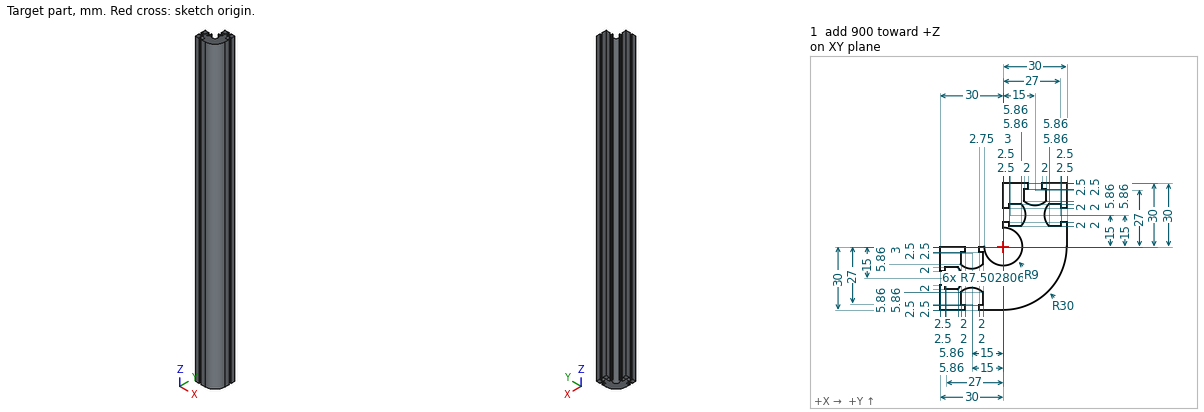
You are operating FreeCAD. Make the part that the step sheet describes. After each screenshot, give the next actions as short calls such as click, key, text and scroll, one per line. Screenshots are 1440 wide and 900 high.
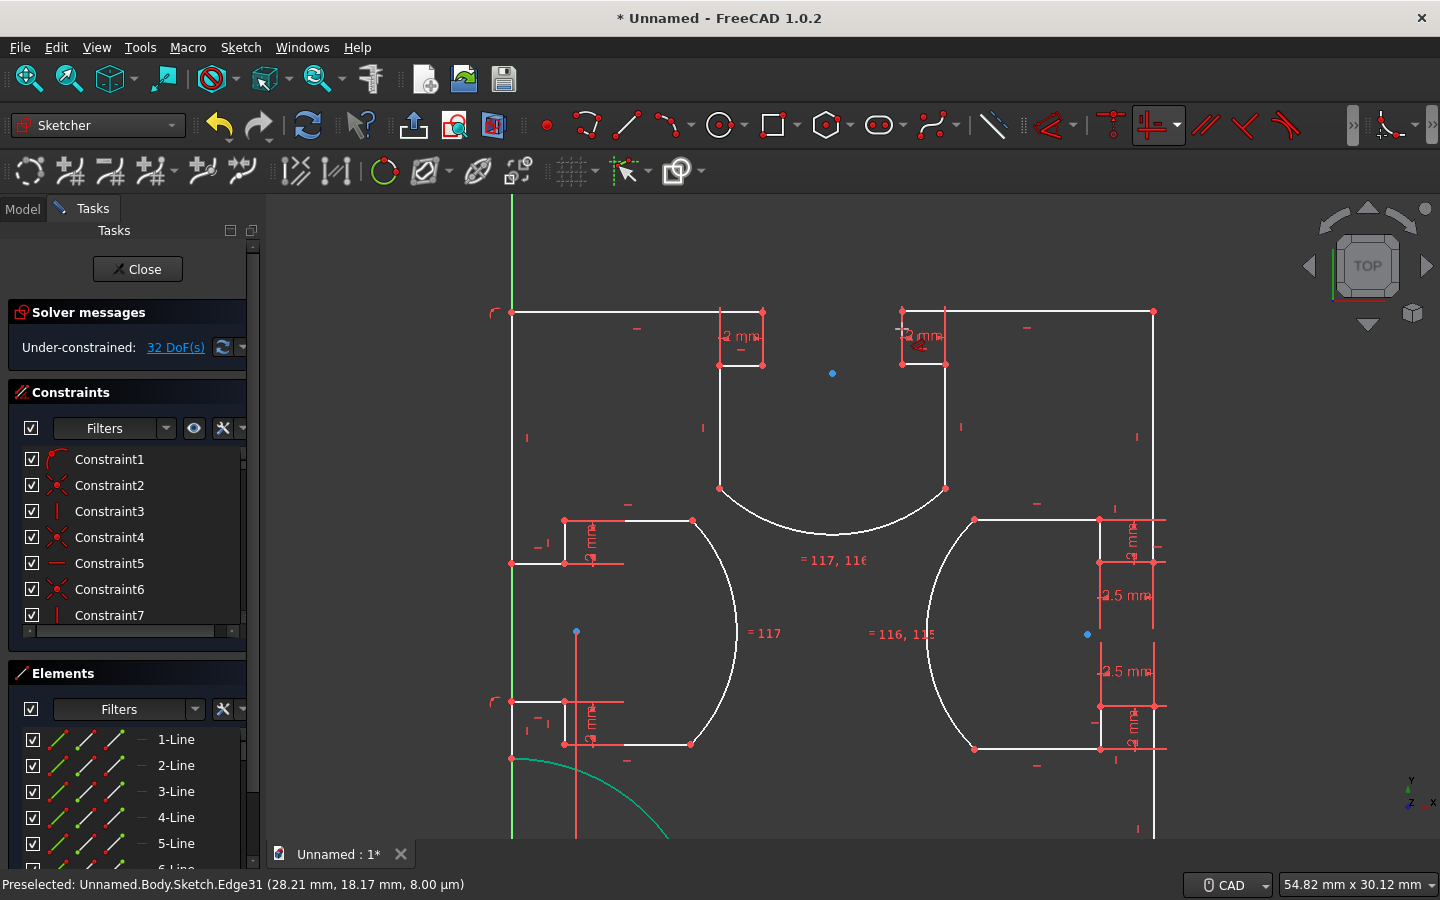
click(902, 327)
click(844, 338)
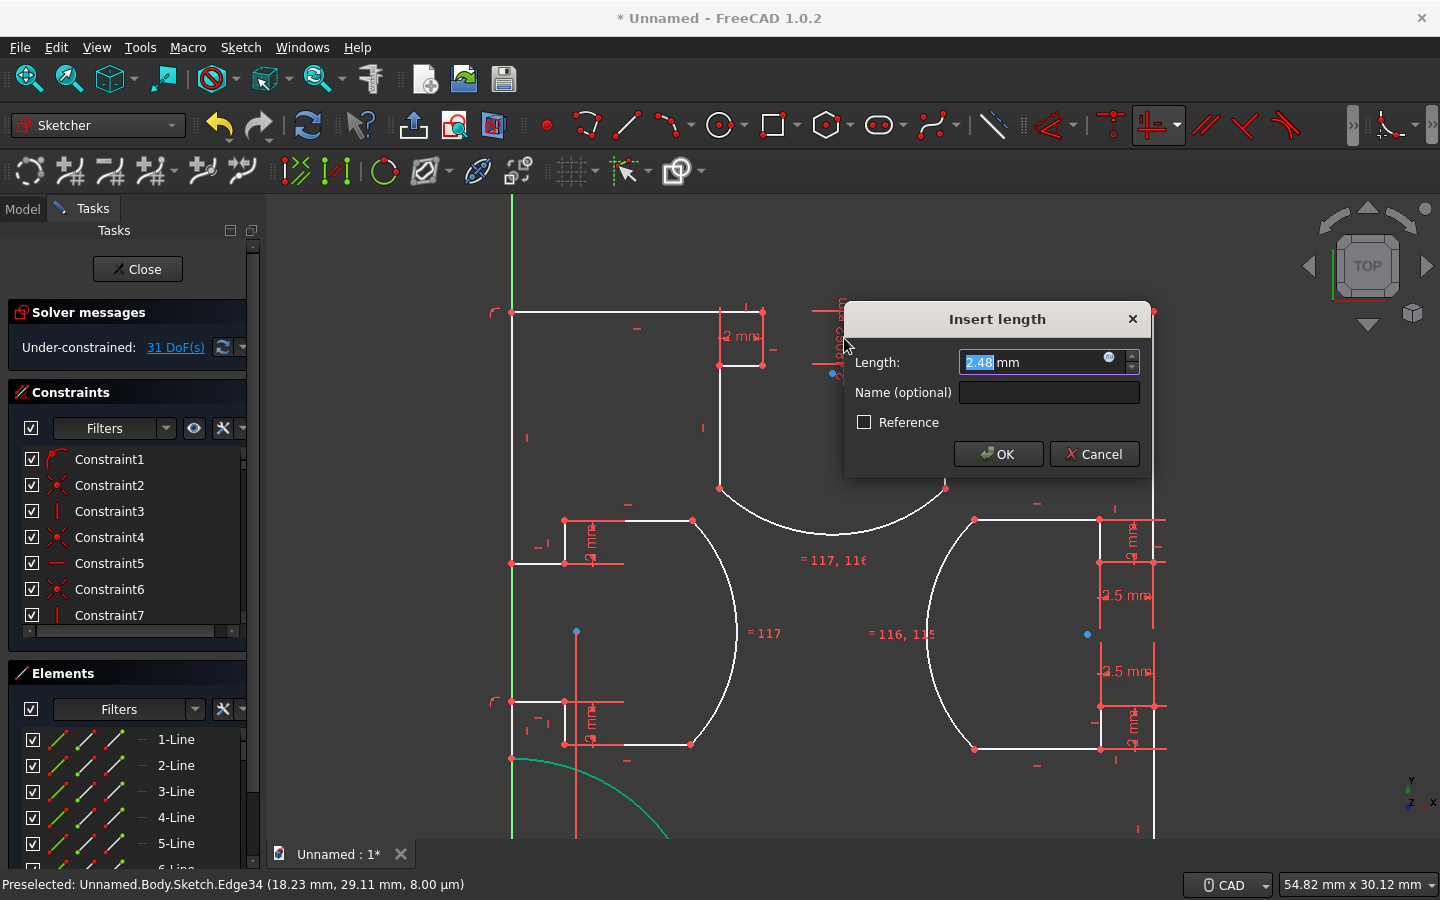
text(2.5)
key(Return)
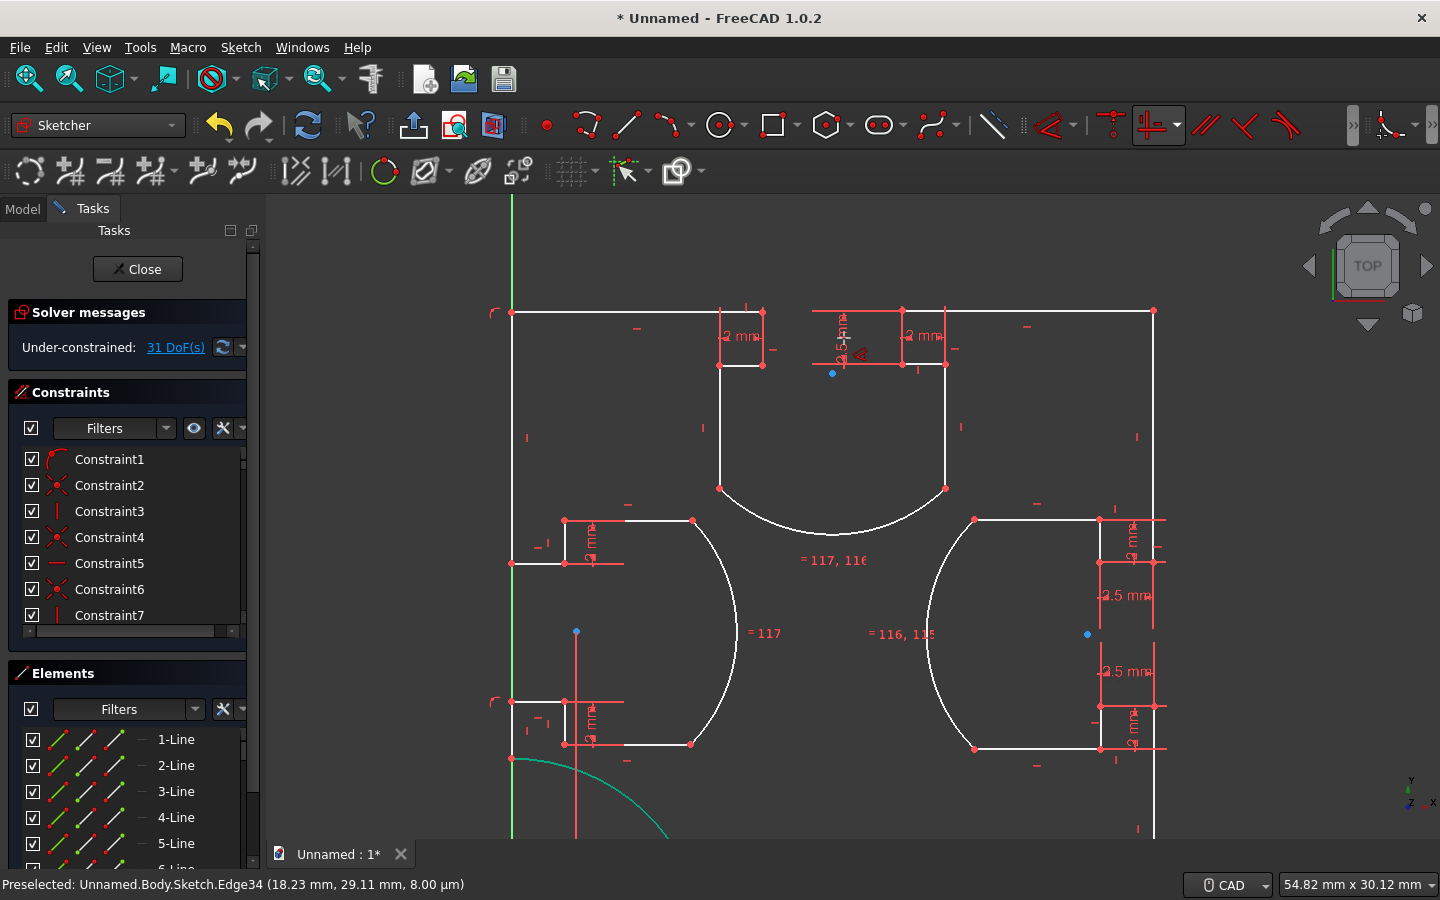
click(763, 350)
click(657, 339)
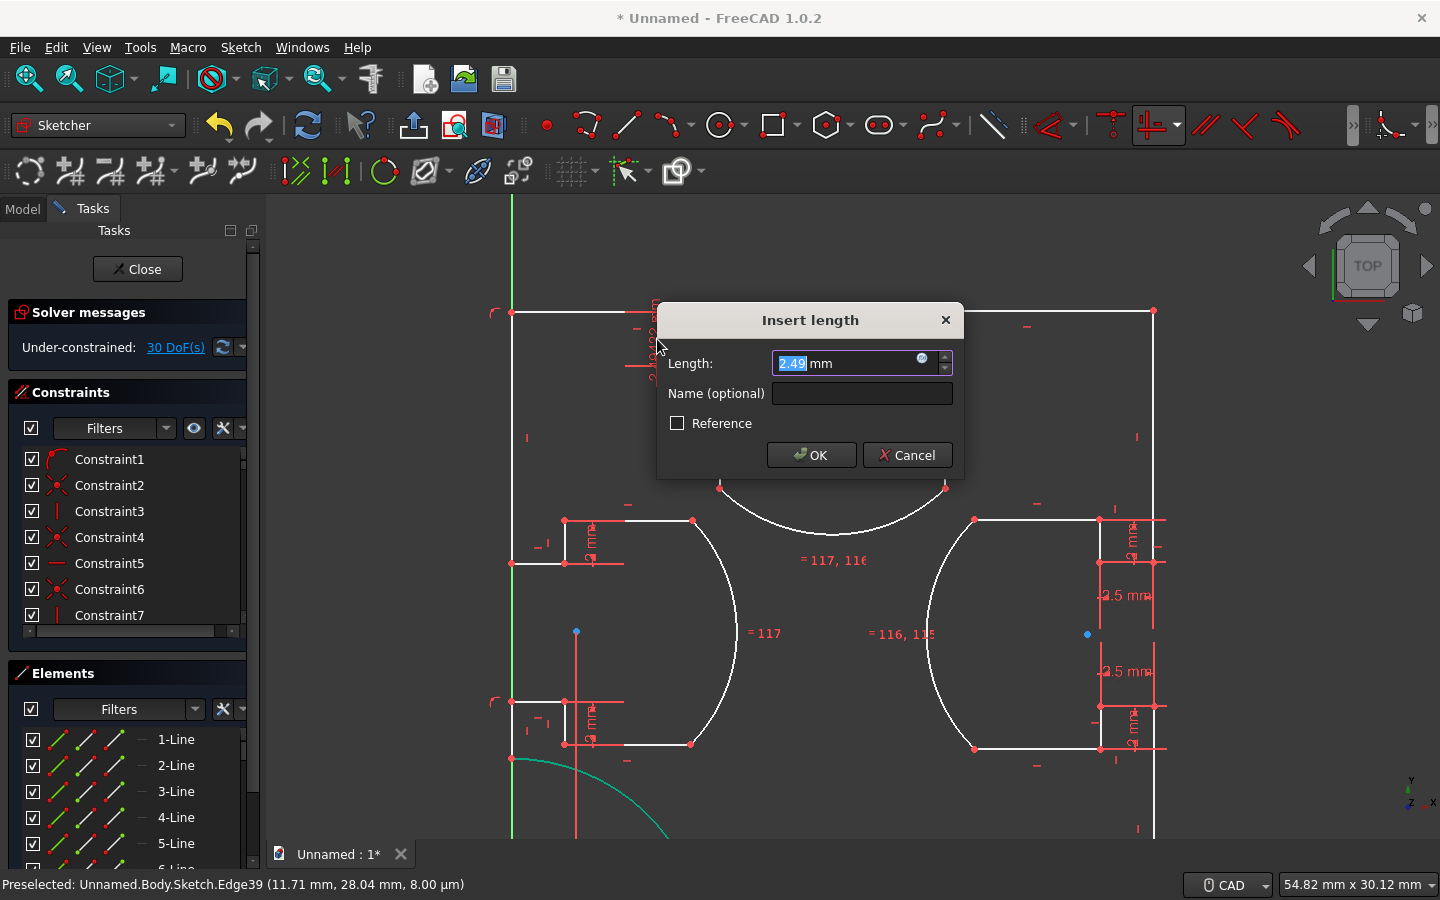
text(2.5)
key(Return)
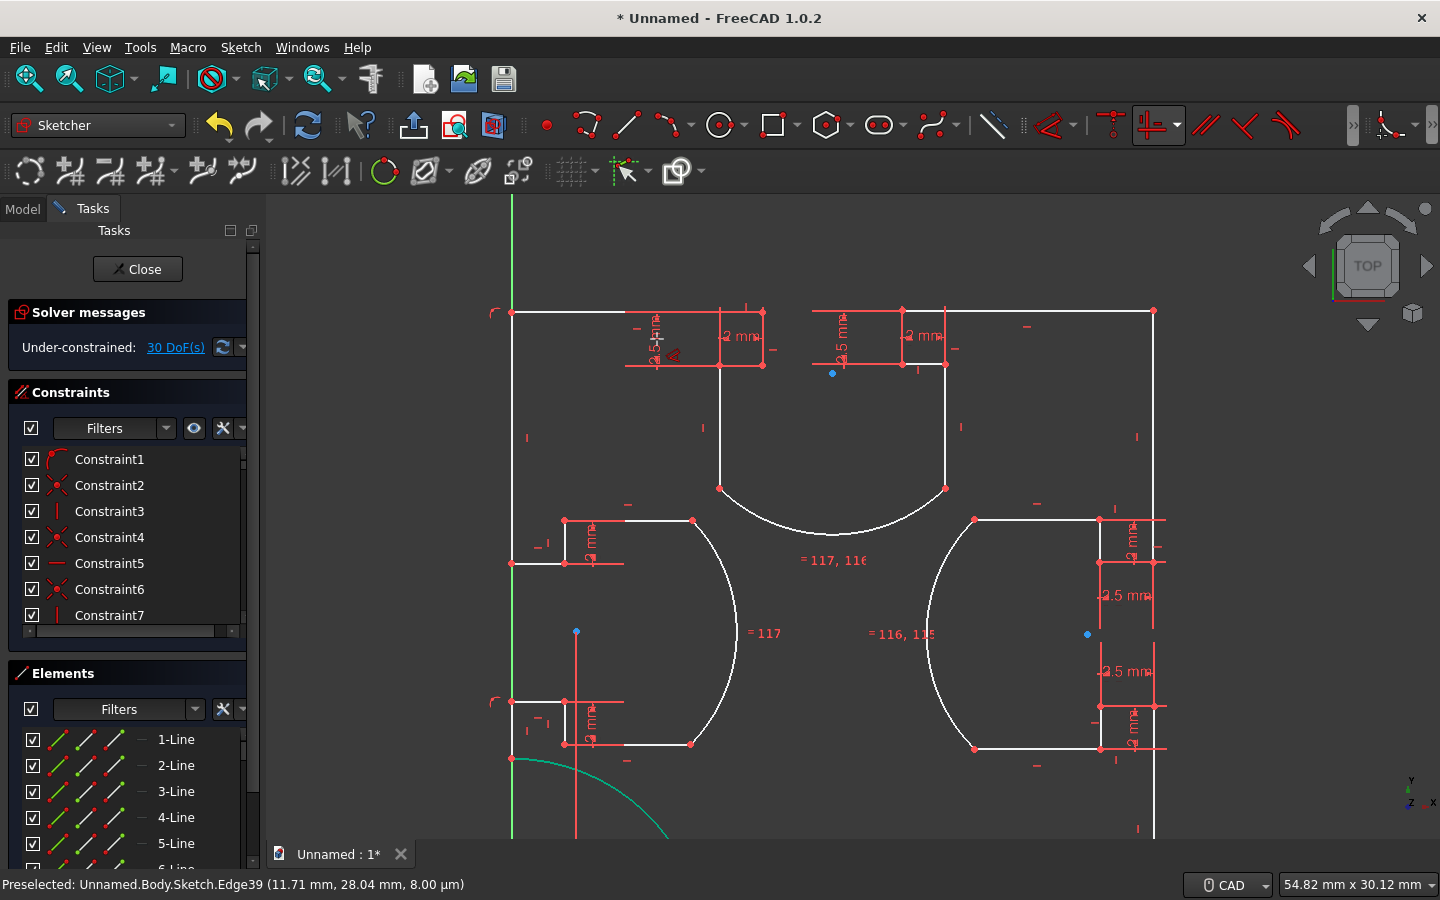
click(528, 564)
click(538, 598)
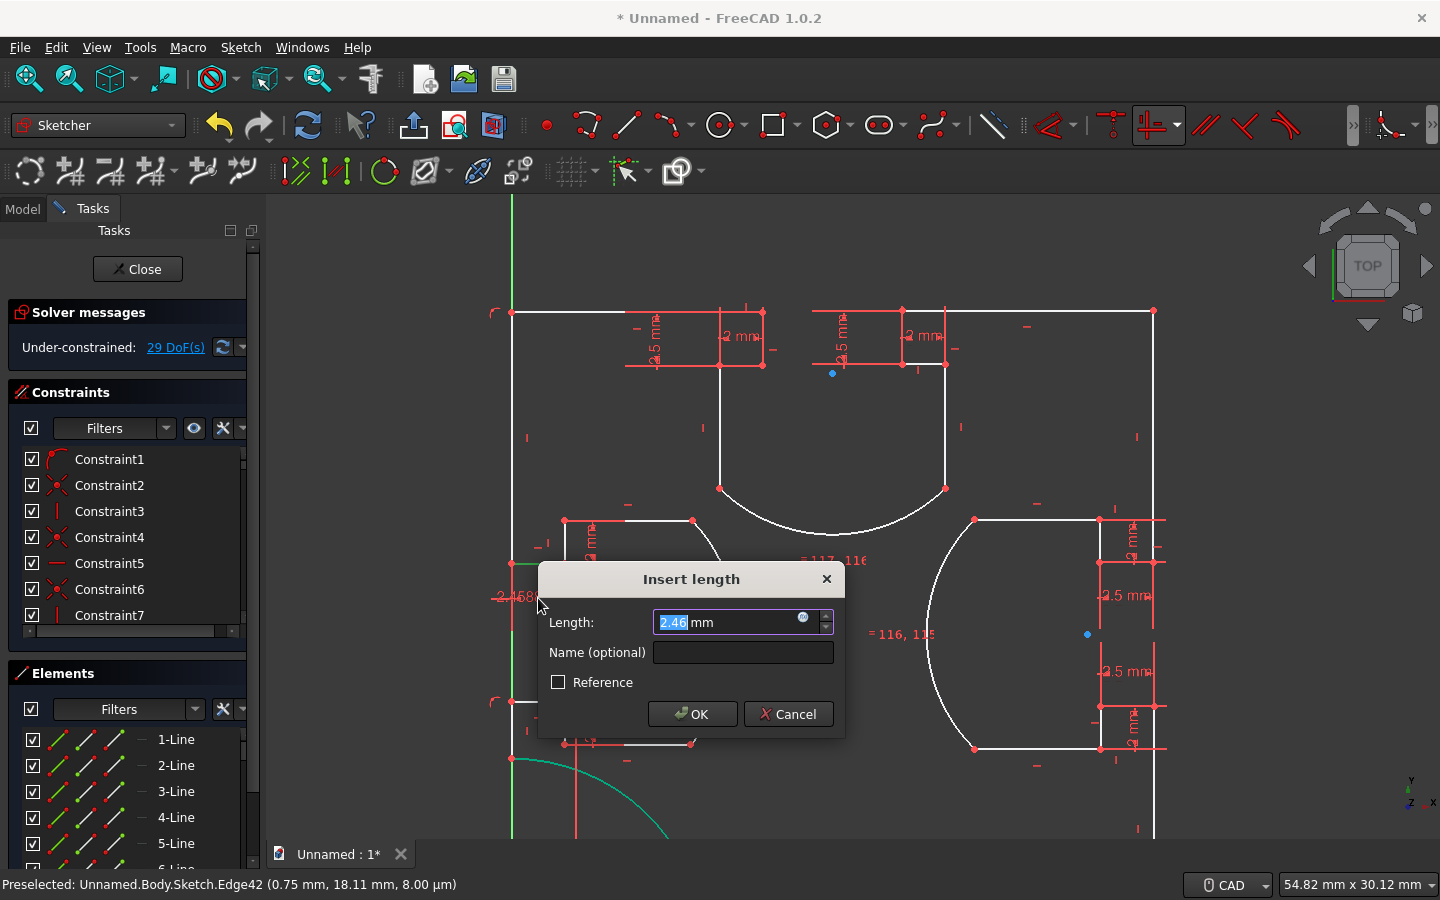
text(2.5)
key(Return)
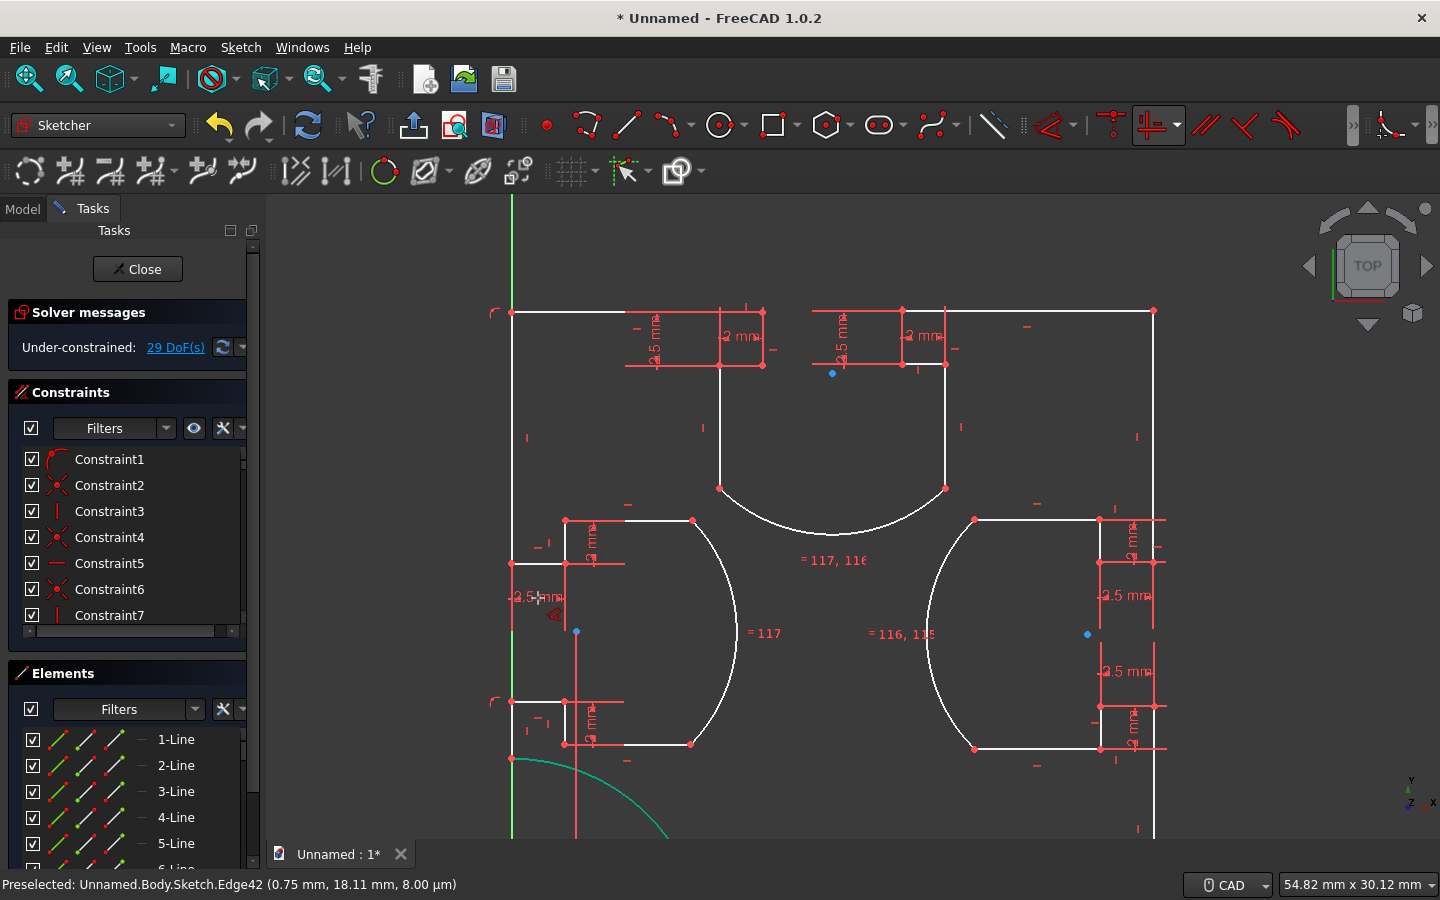
click(549, 702)
click(538, 668)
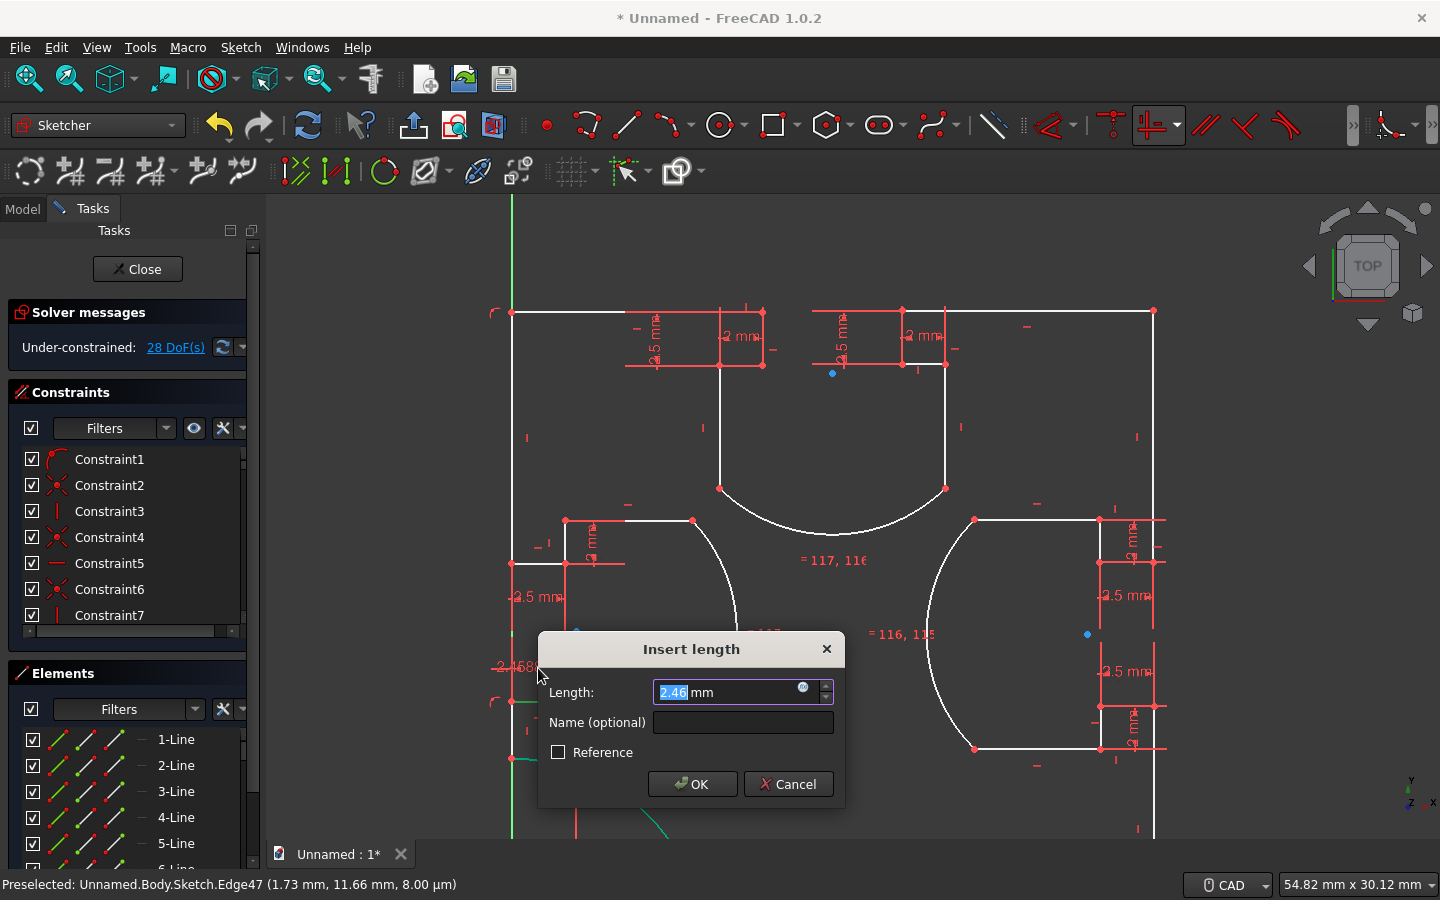
text(2.5)
key(Return)